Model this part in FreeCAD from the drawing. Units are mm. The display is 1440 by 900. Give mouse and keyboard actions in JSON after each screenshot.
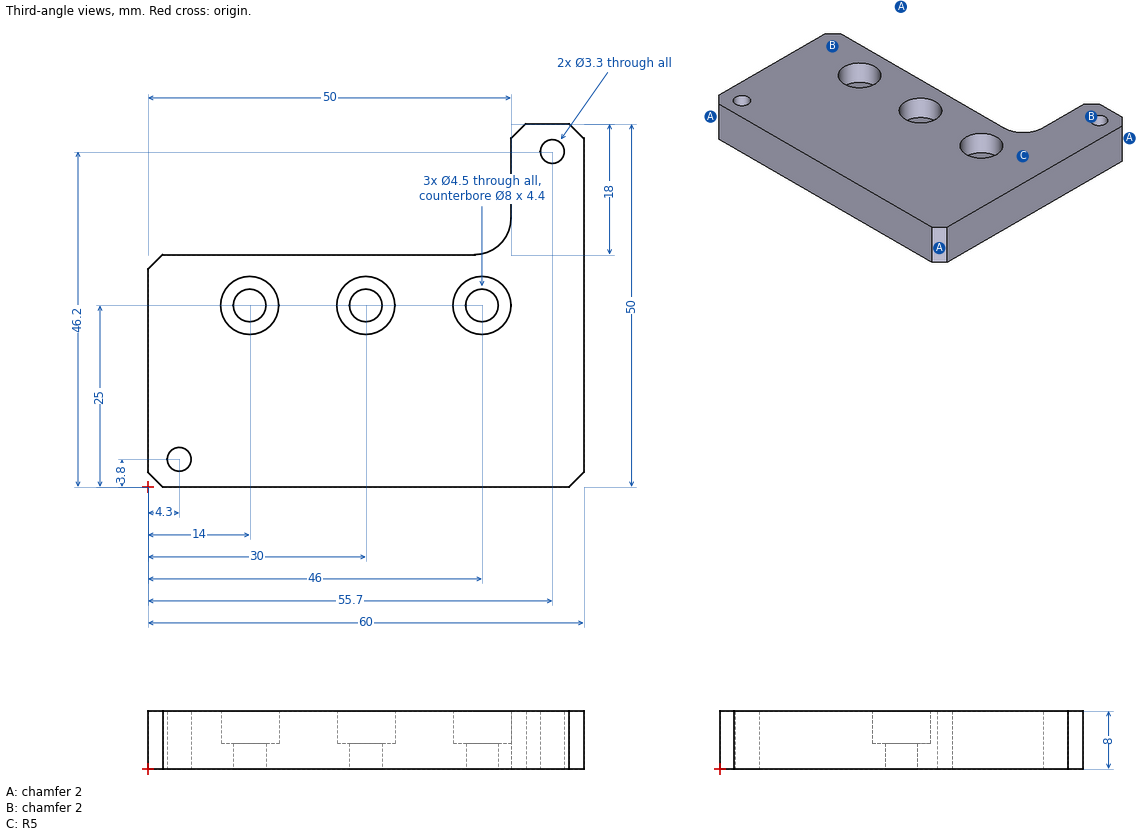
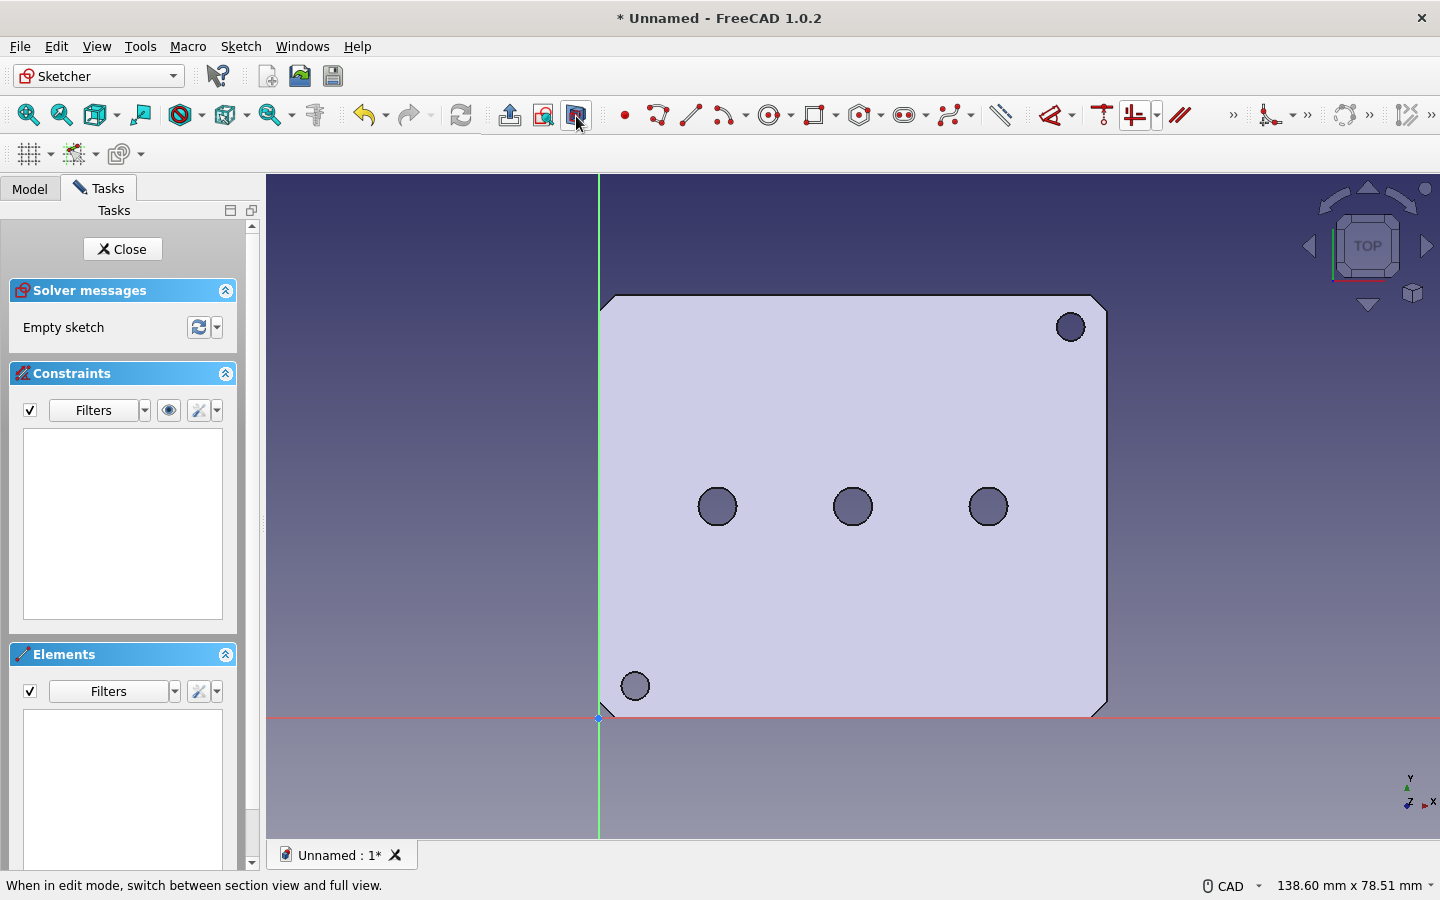
{"action": "left_click", "coordinate": [814, 116]}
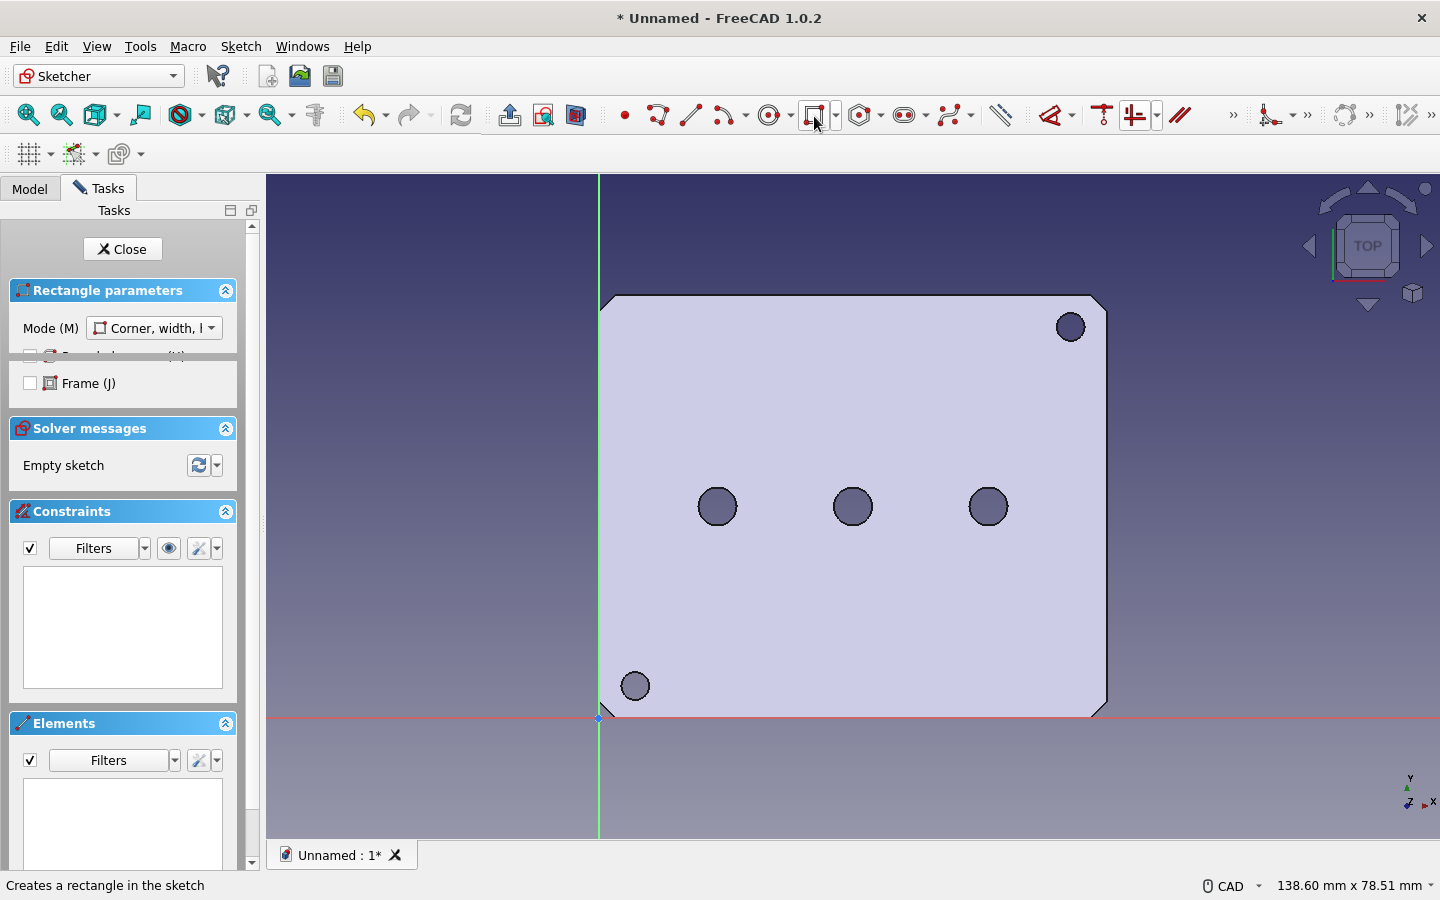
{"action": "left_click", "coordinate": [599, 295]}
{"action": "mouse_move", "coordinate": [1022, 447]}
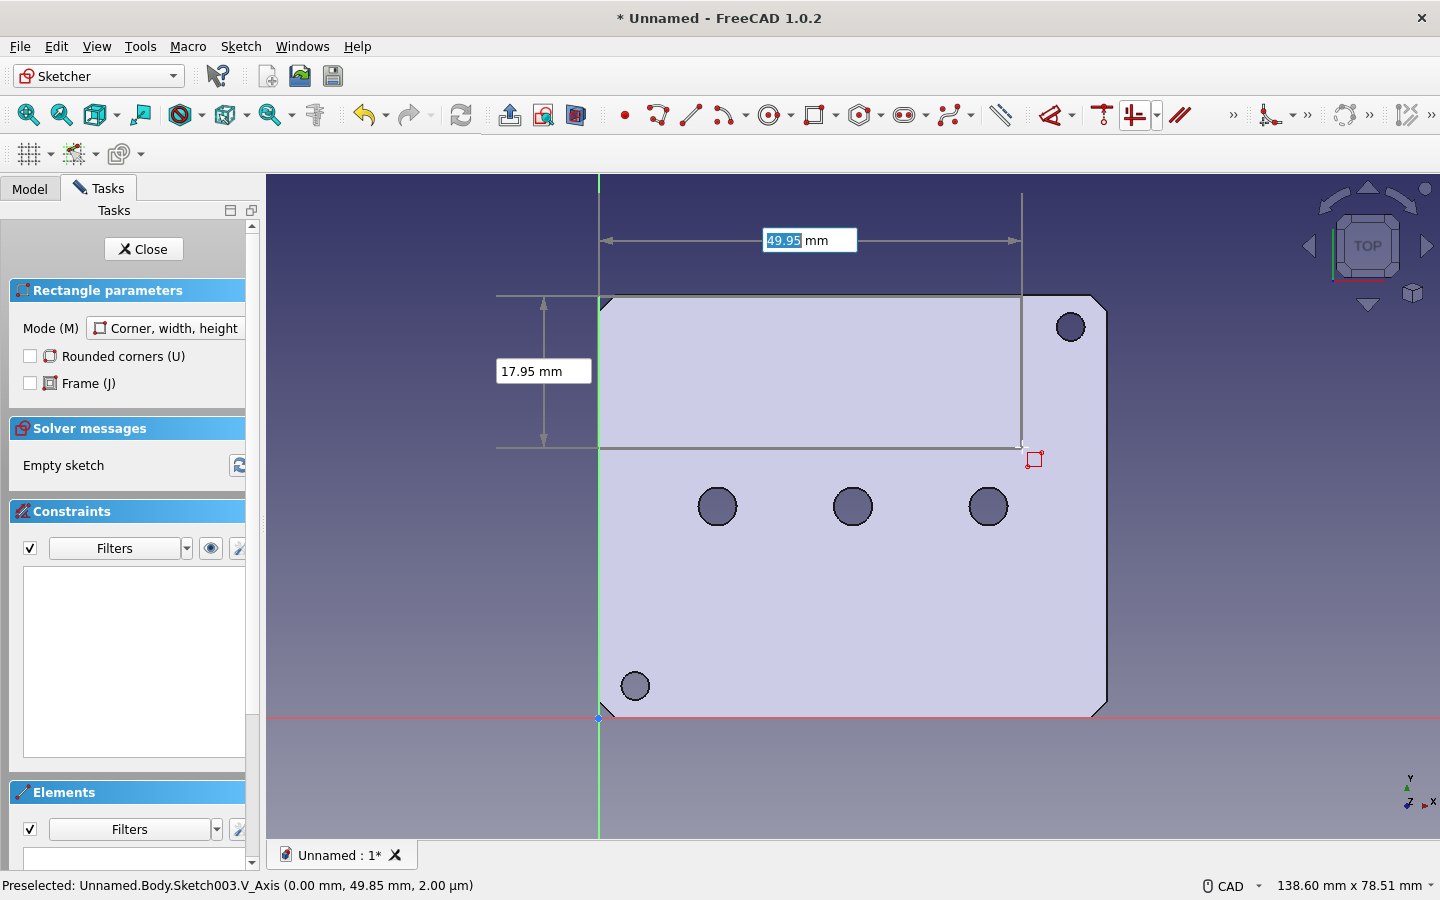
{"action": "type", "text": "50"}
{"action": "key", "text": "Tab"}
{"action": "type", "text": "18"}
{"action": "key", "text": "Return"}
{"action": "key", "text": "Escape"}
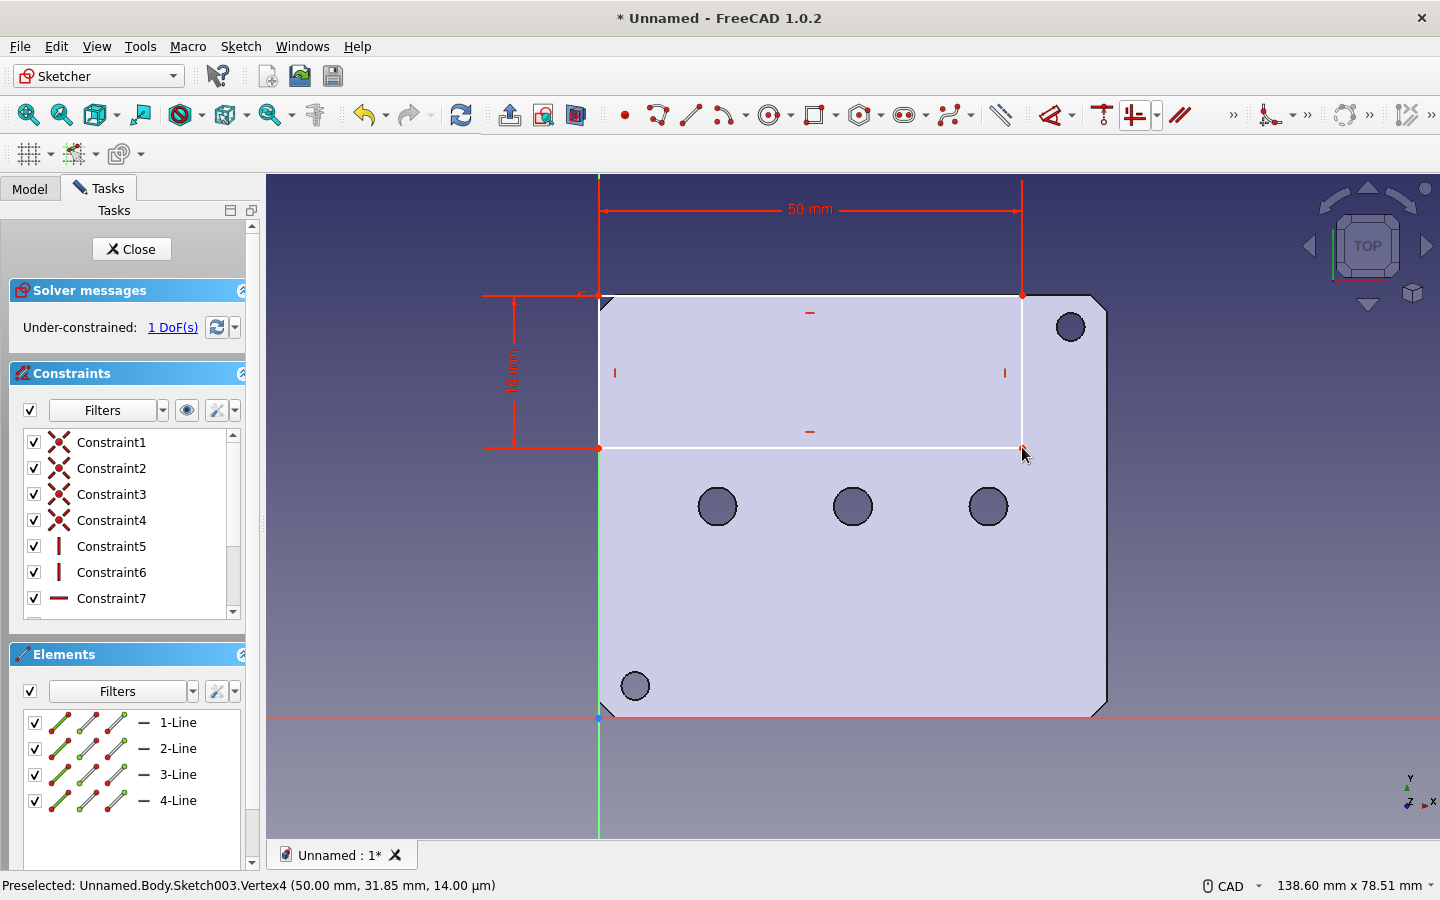
{"action": "left_click", "coordinate": [1050, 116]}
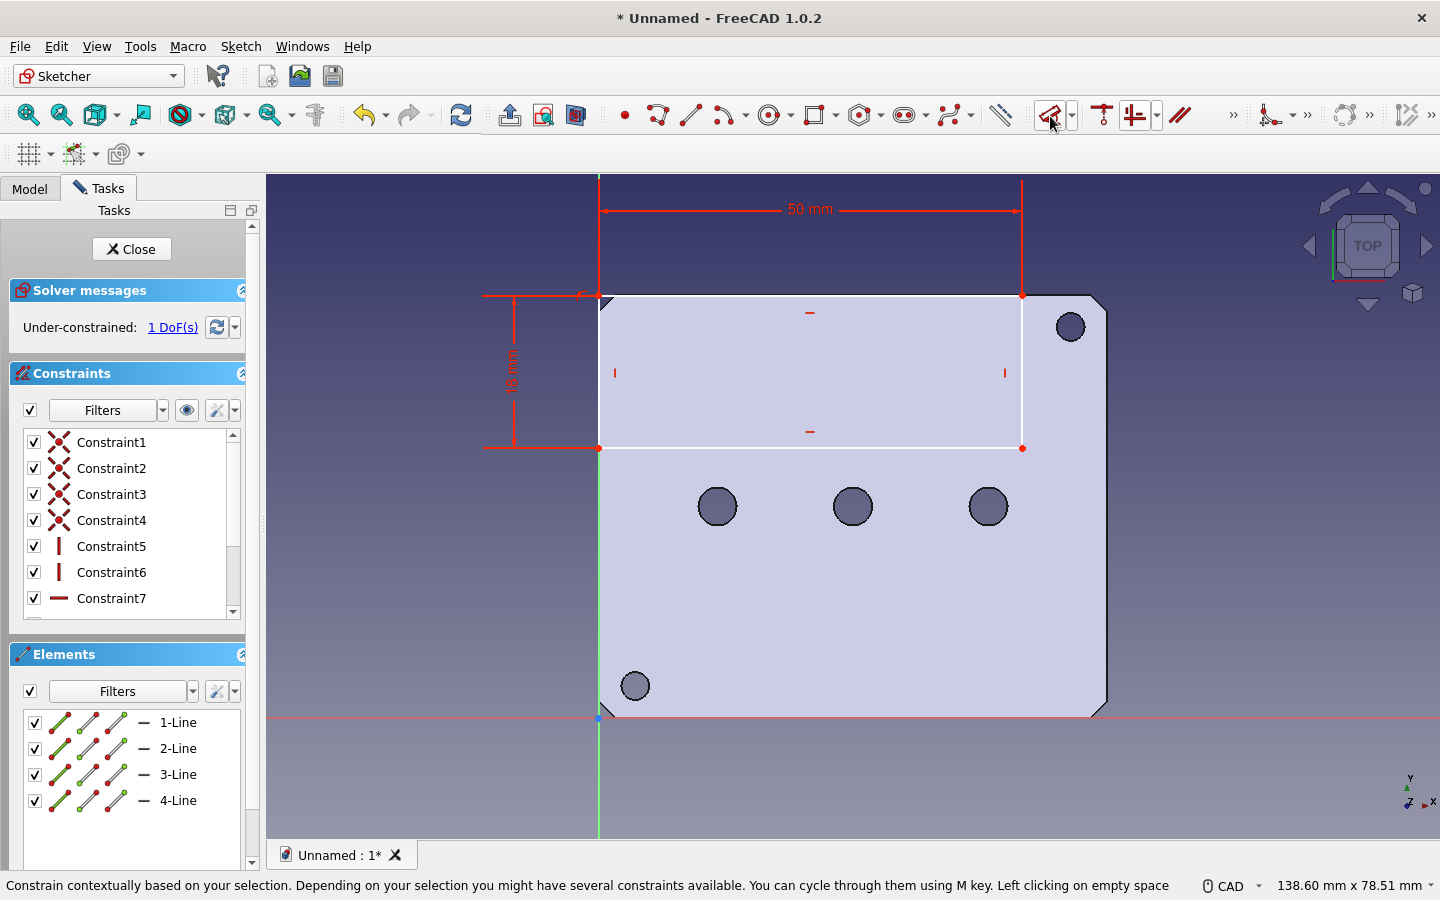
{"action": "left_click", "coordinate": [599, 296]}
{"action": "left_click", "coordinate": [565, 507]}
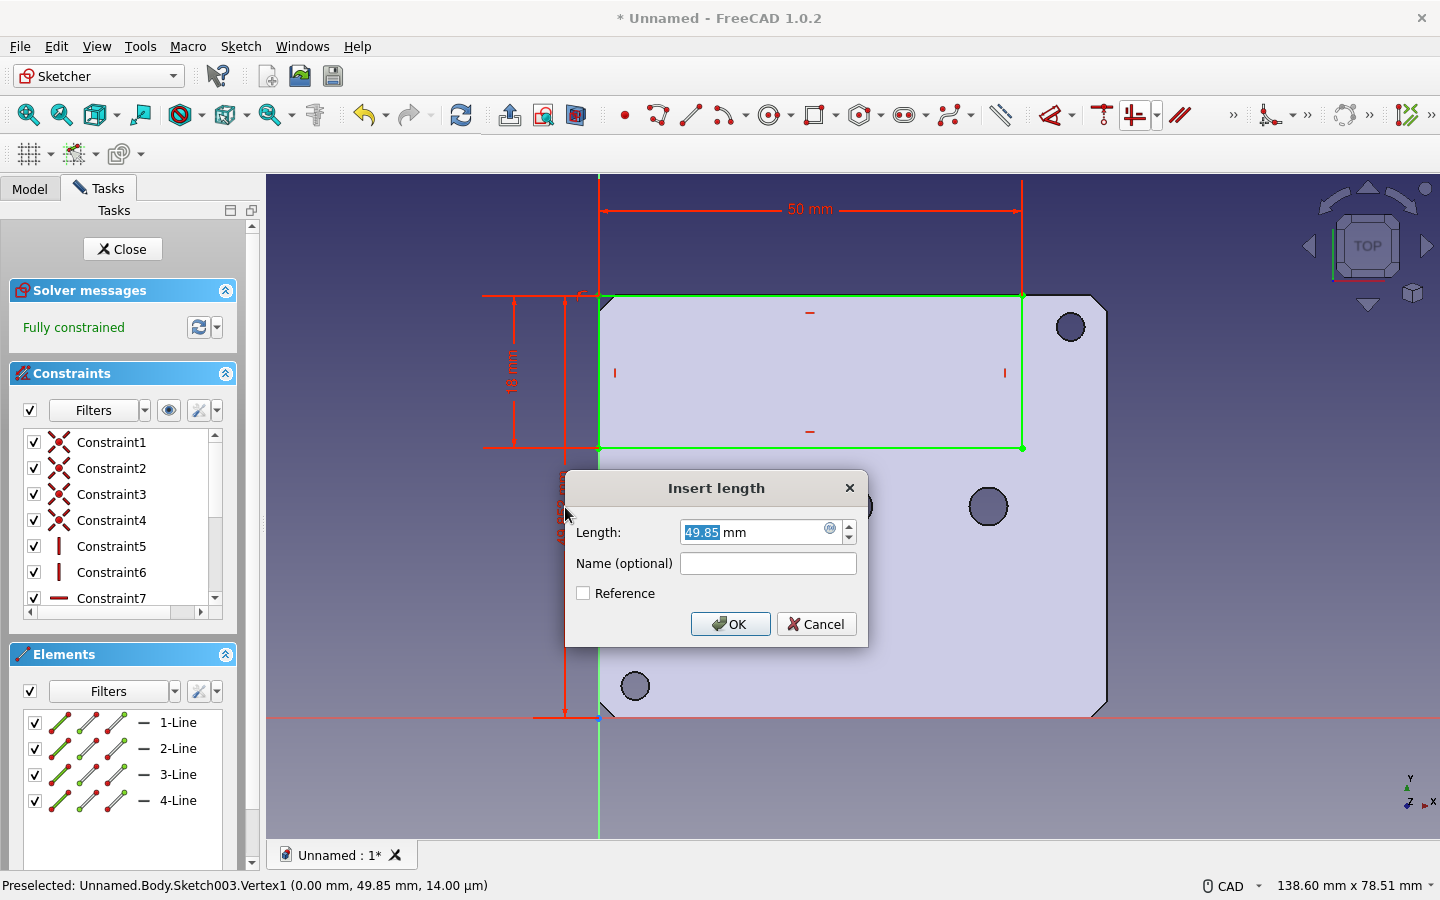
{"action": "type", "text": "50"}
{"action": "key", "text": "Return"}
{"action": "key", "text": "Escape"}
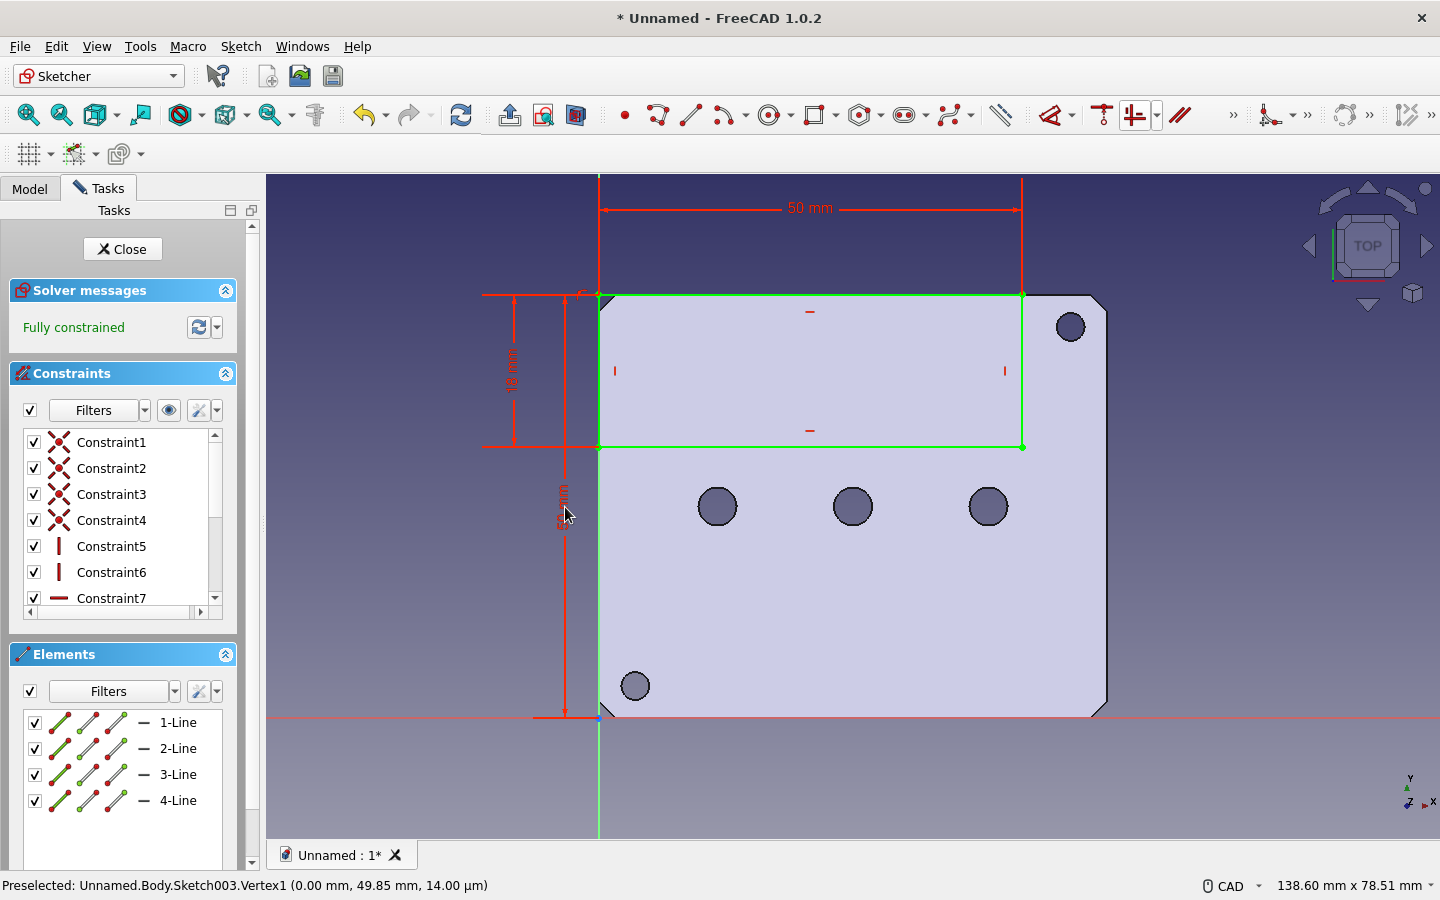
{"action": "left_click", "coordinate": [123, 249]}